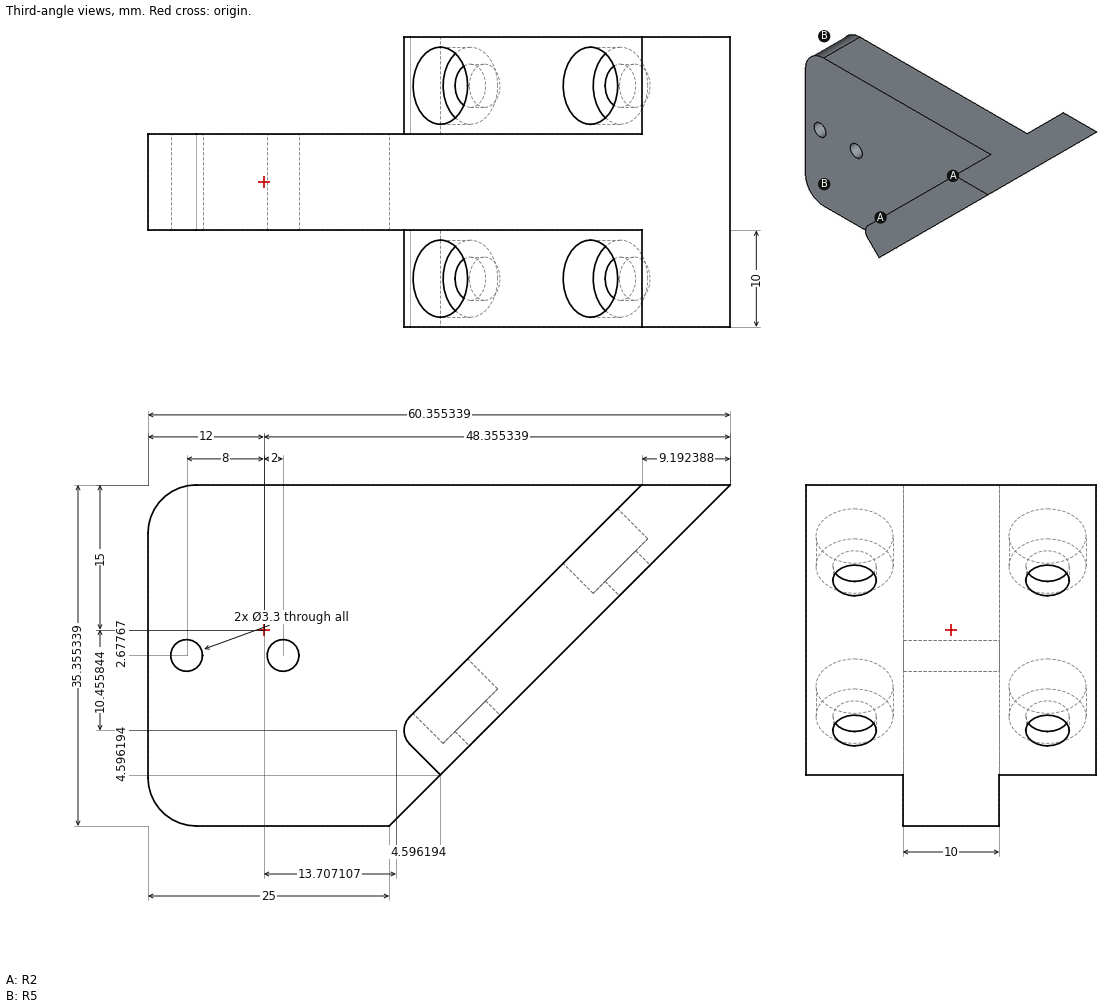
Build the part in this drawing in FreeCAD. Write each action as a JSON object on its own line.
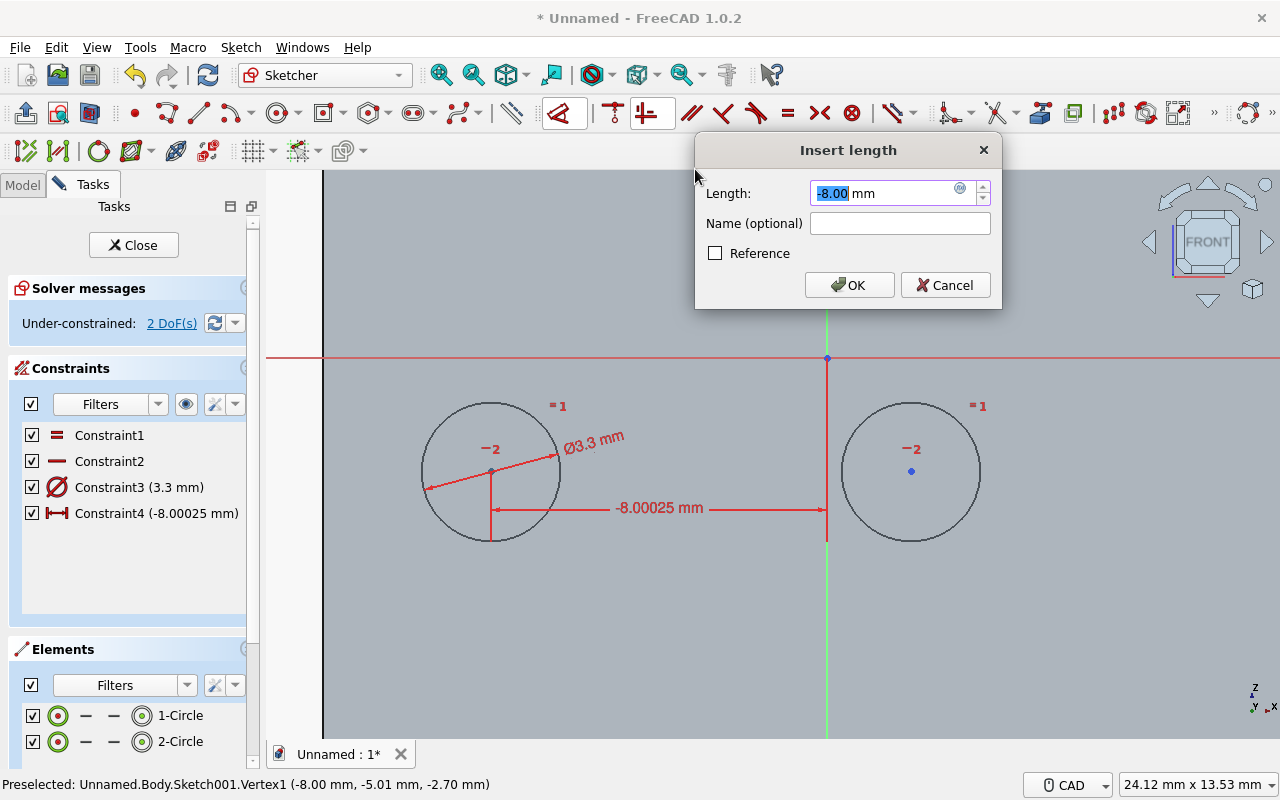
{"action": "type", "text": "-8"}
{"action": "key", "text": "Return"}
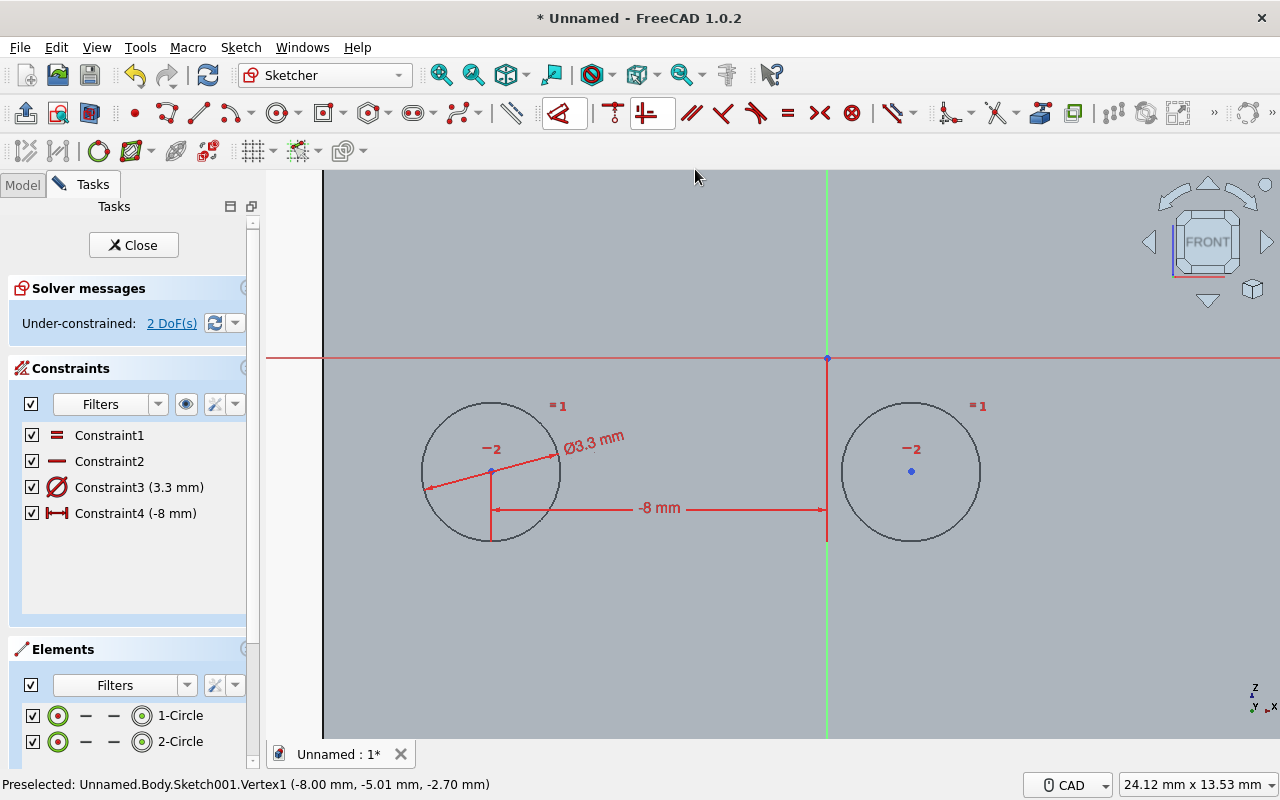
{"action": "left_click", "coordinate": [911, 472]}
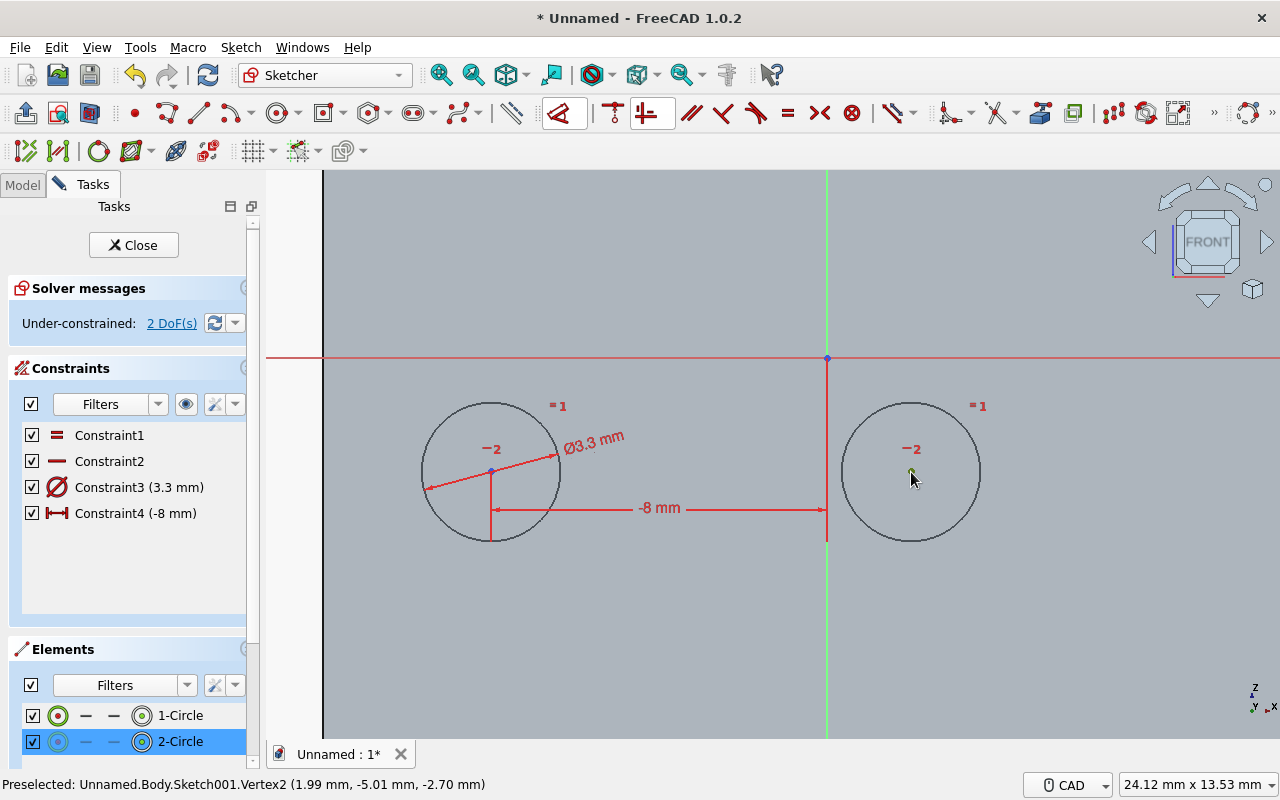
{"action": "left_click", "coordinate": [582, 114]}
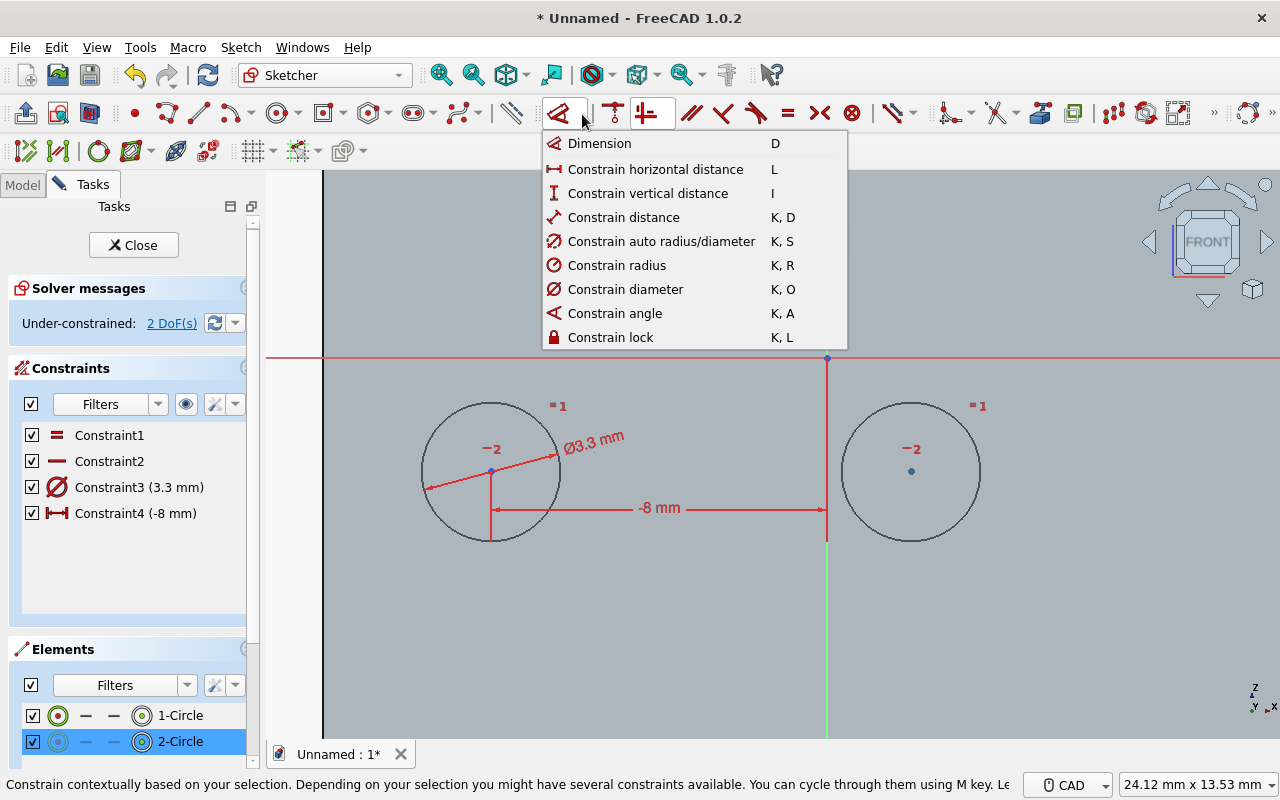
{"action": "left_click", "coordinate": [695, 169]}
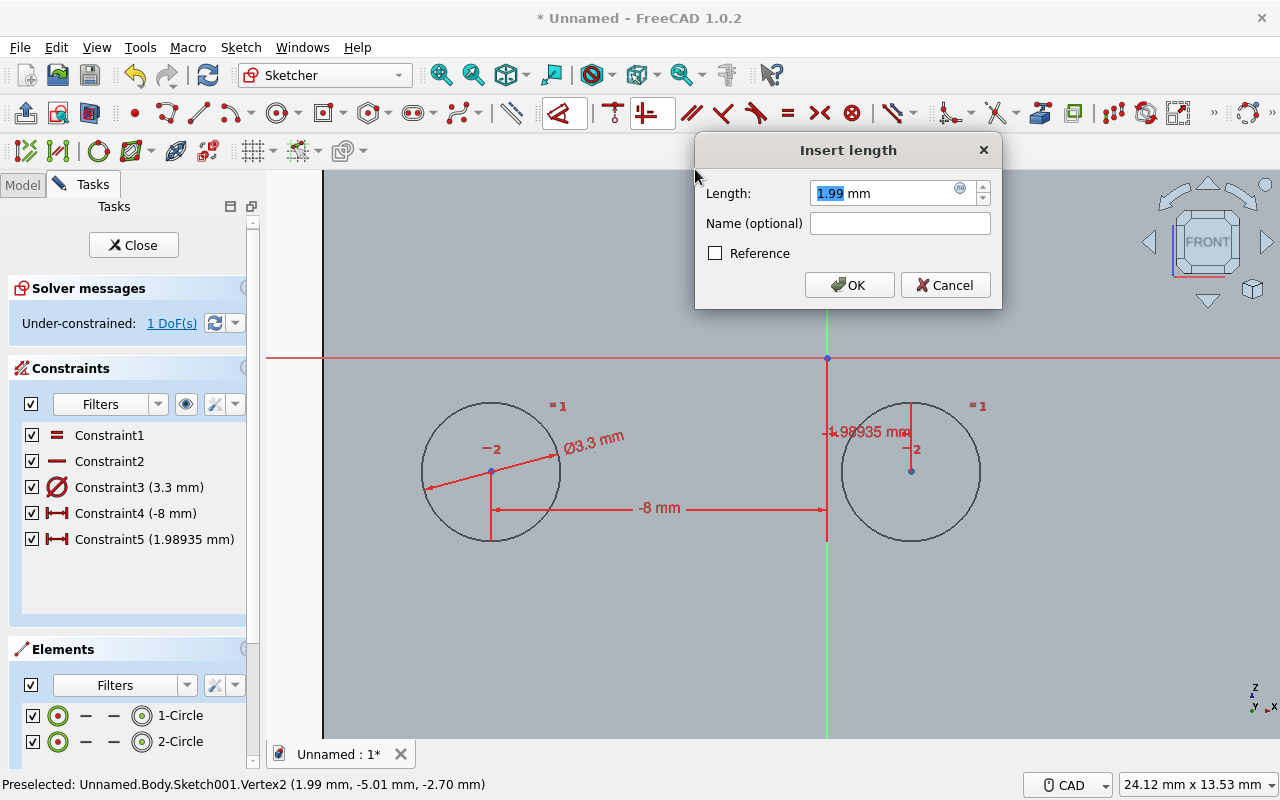
{"action": "type", "text": "2"}
{"action": "key", "text": "Return"}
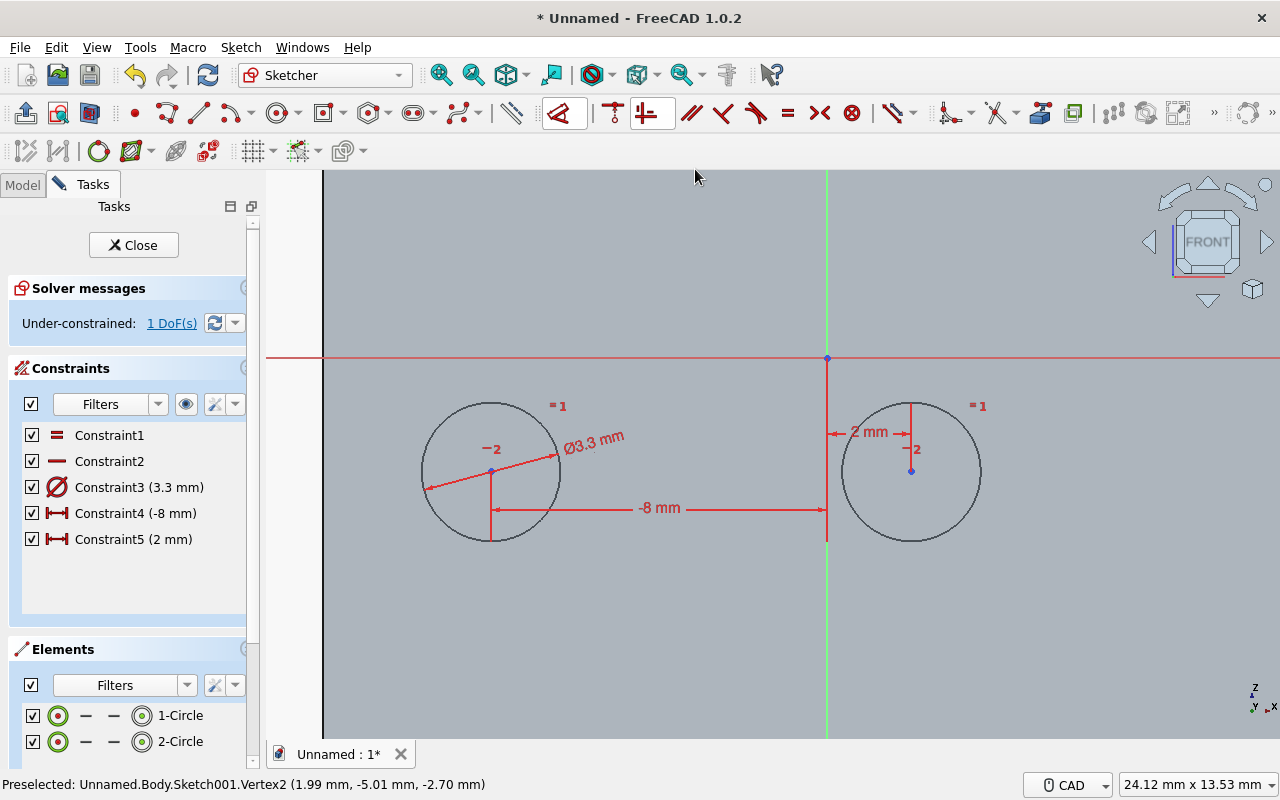
{"action": "left_click", "coordinate": [491, 472]}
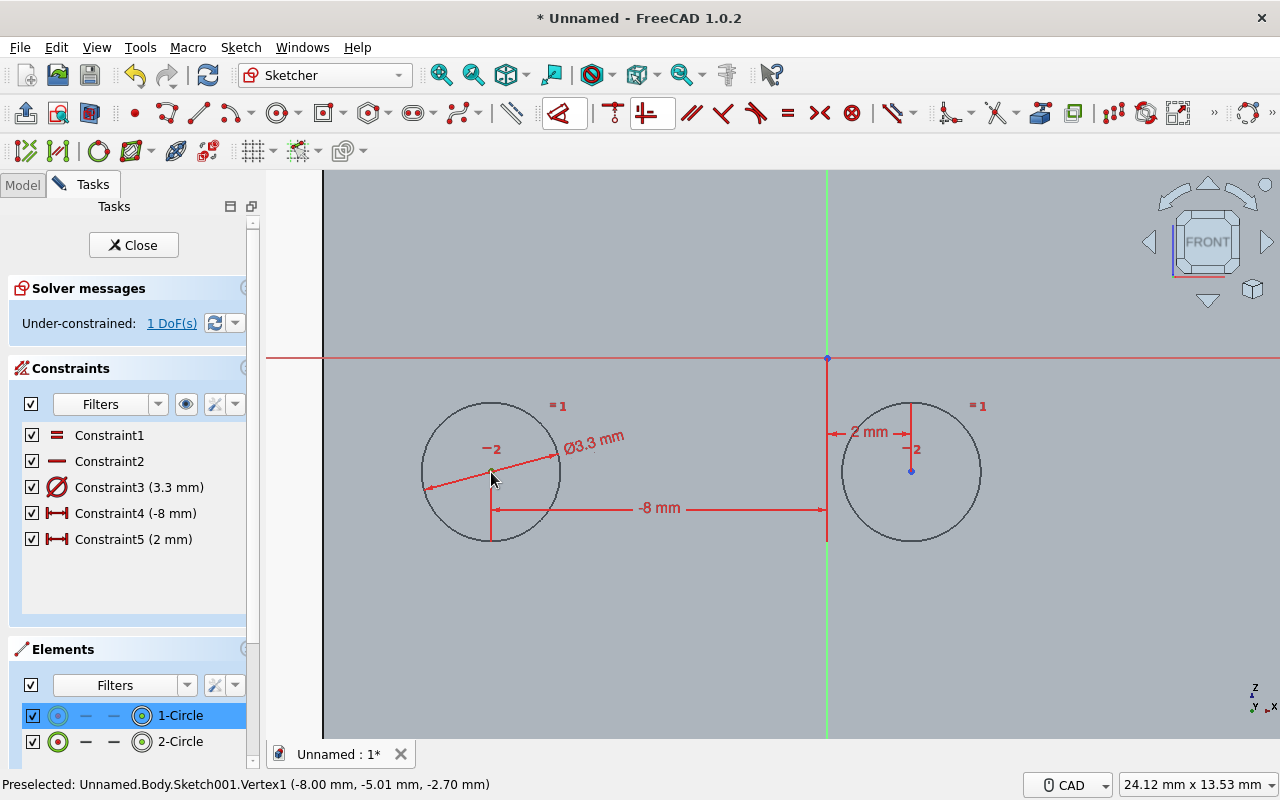
{"action": "key", "text": "i"}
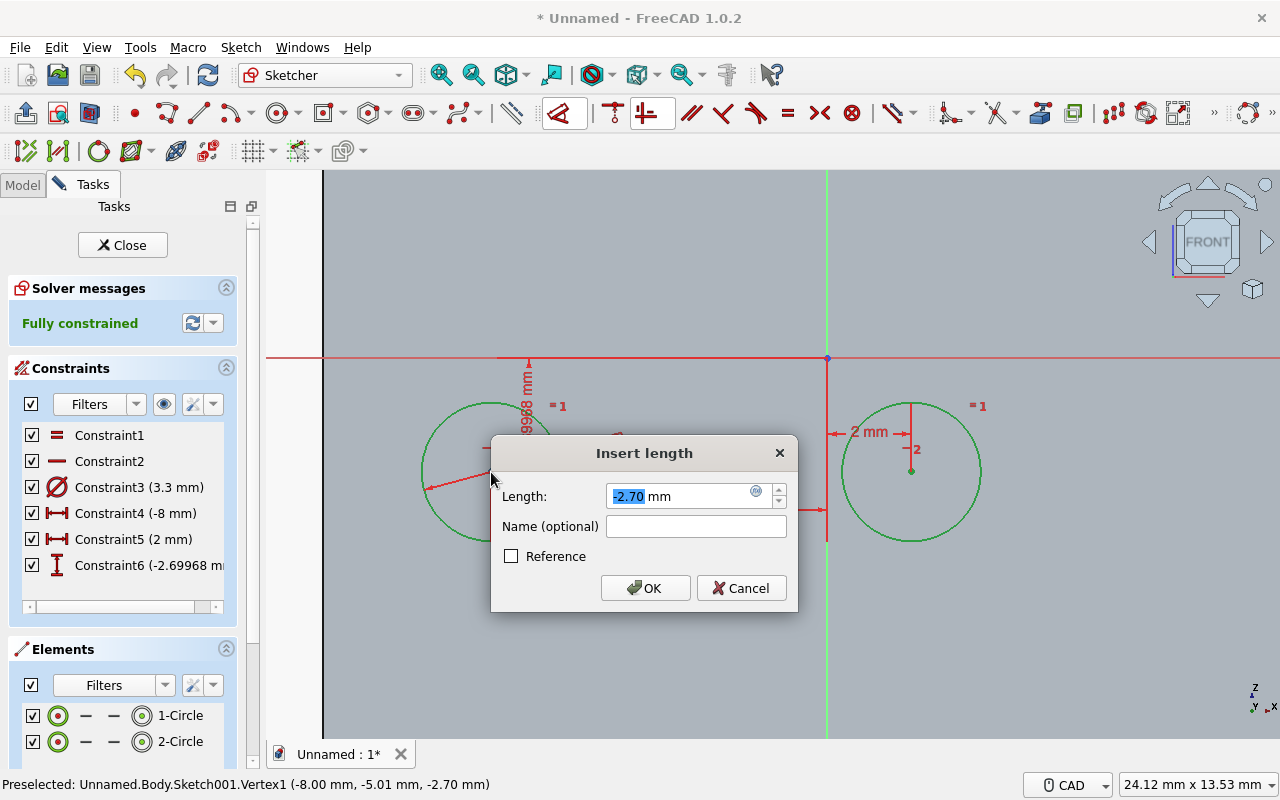
{"action": "type", "text": "-2.67767"}
{"action": "key", "text": "Return"}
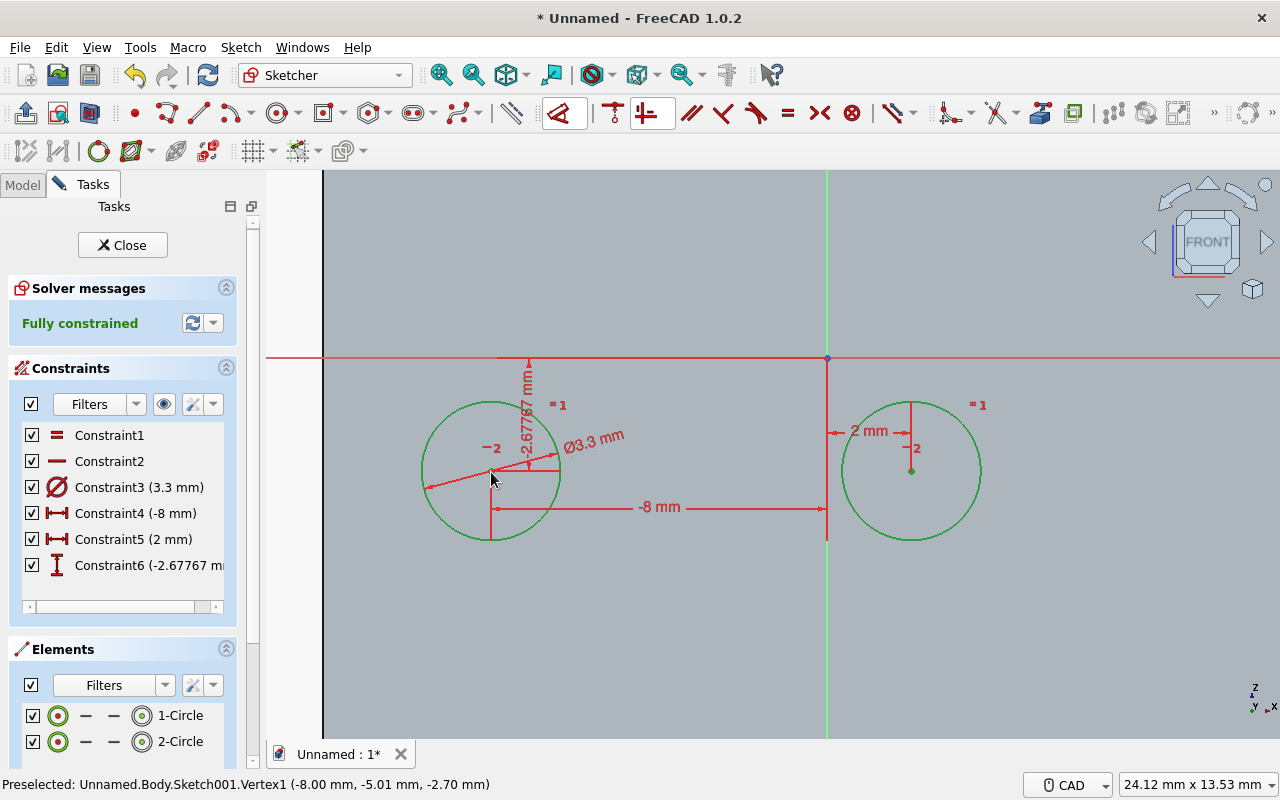
{"action": "left_click", "coordinate": [123, 245]}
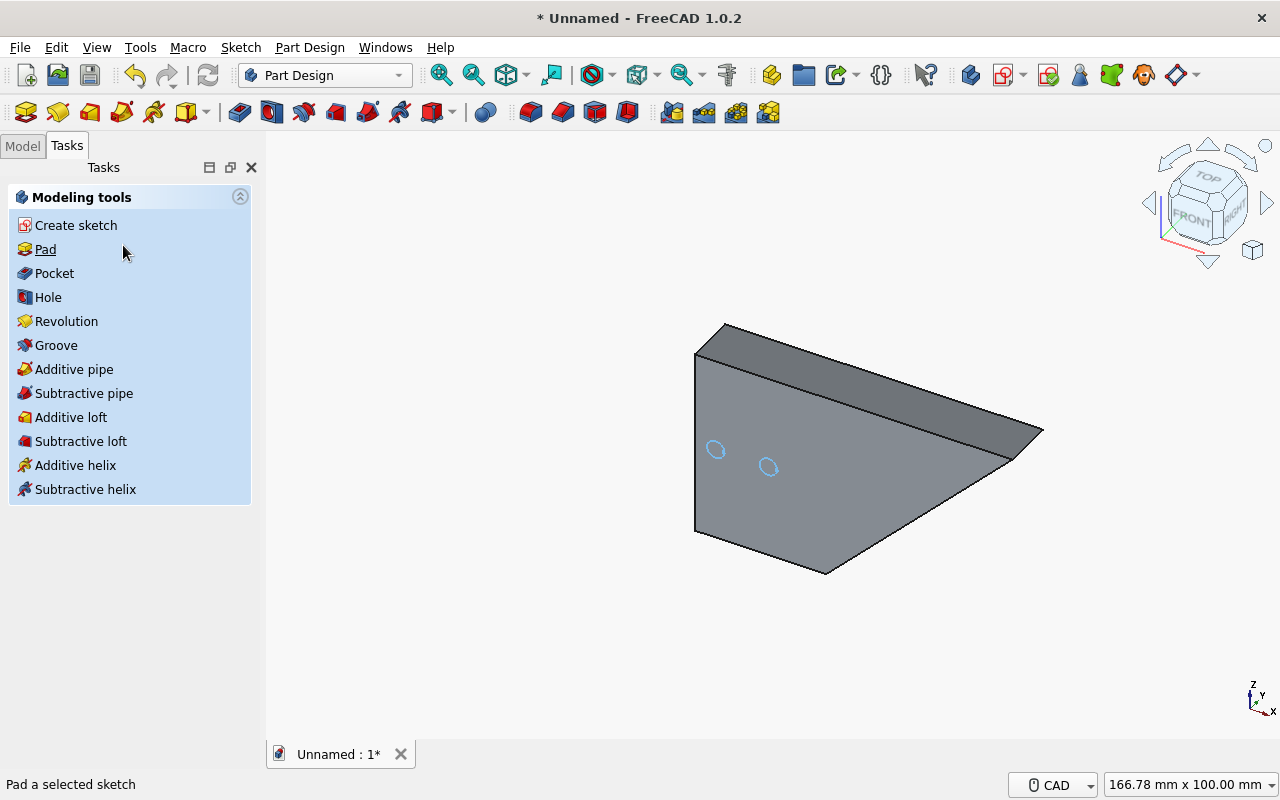
{"action": "left_click", "coordinate": [272, 112]}